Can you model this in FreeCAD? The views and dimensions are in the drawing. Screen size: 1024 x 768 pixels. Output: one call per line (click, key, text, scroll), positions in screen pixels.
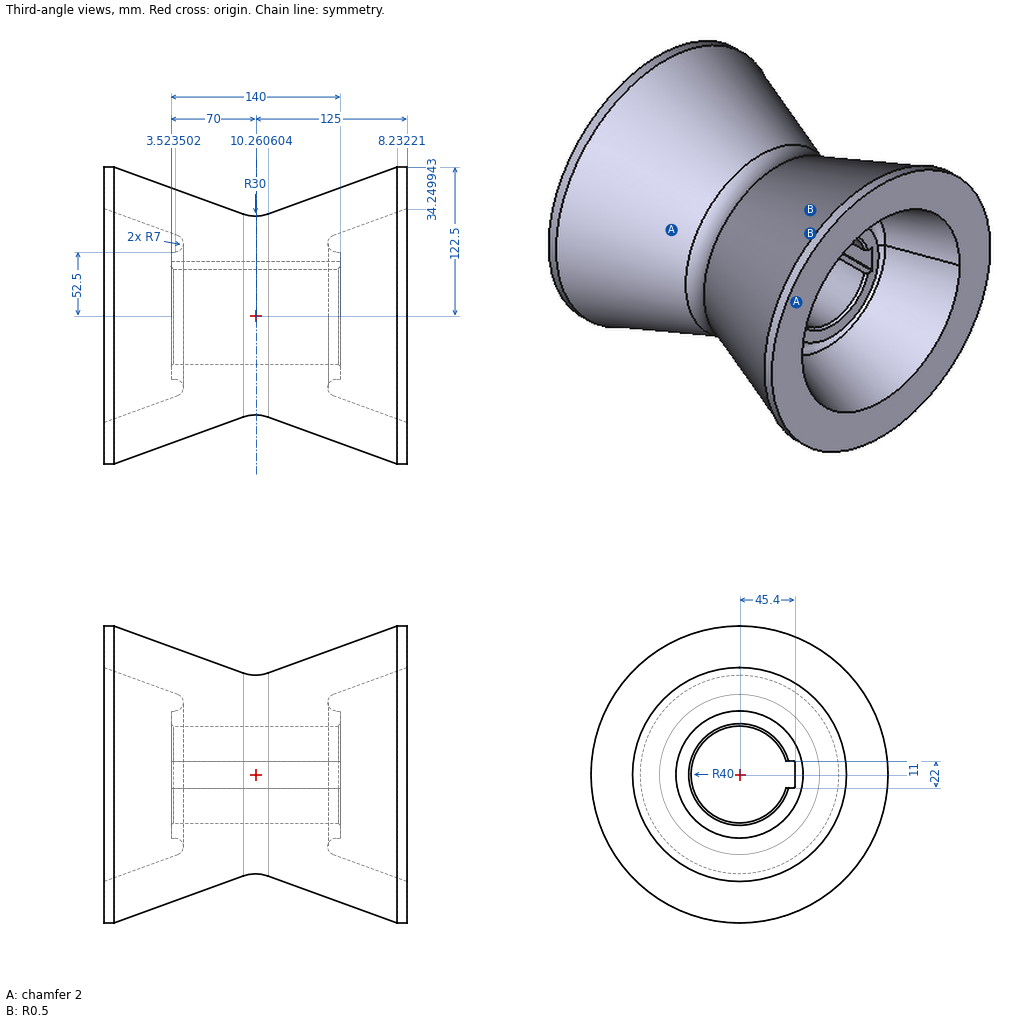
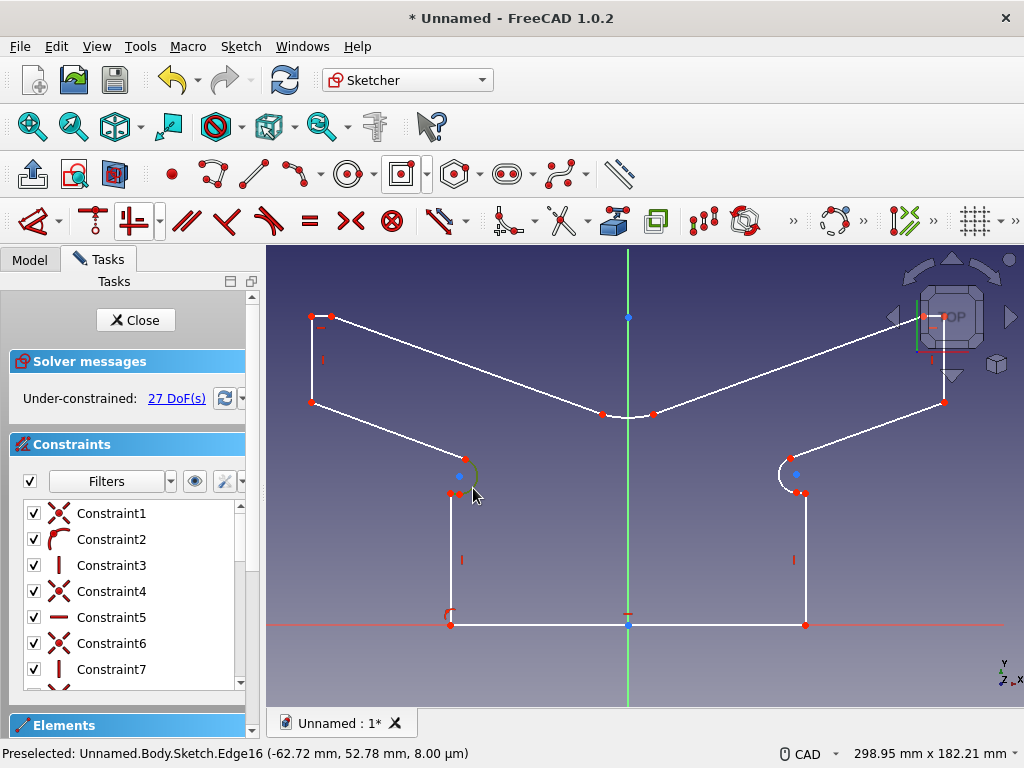
click(269, 222)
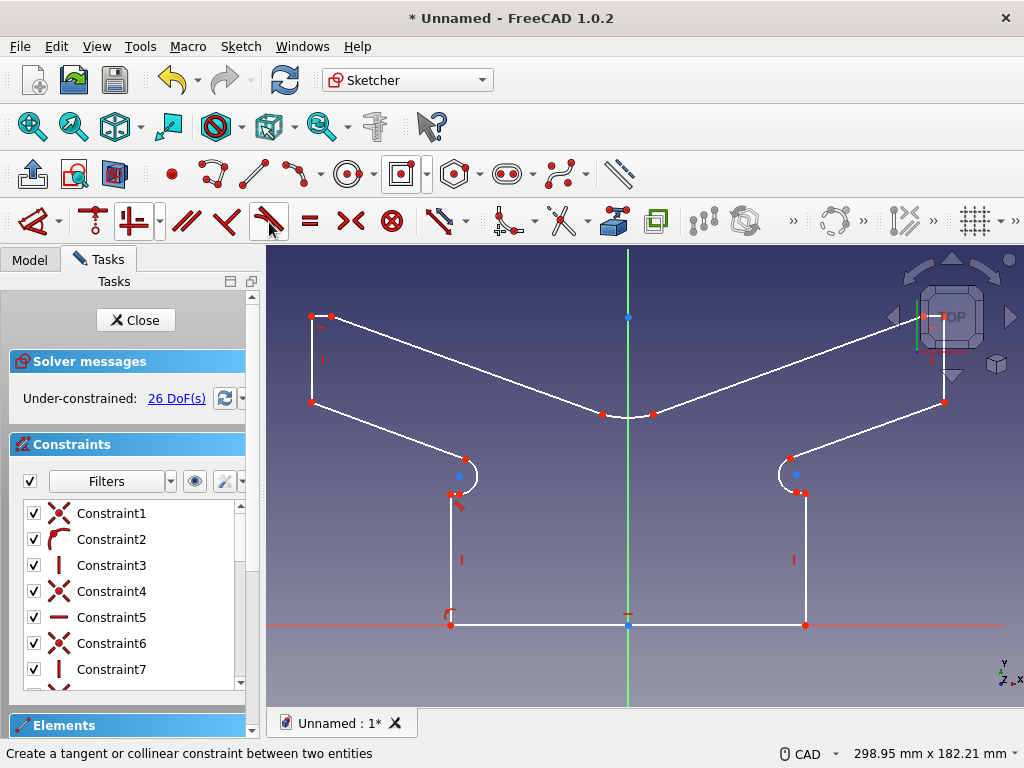
scroll(801, 493, up, 6)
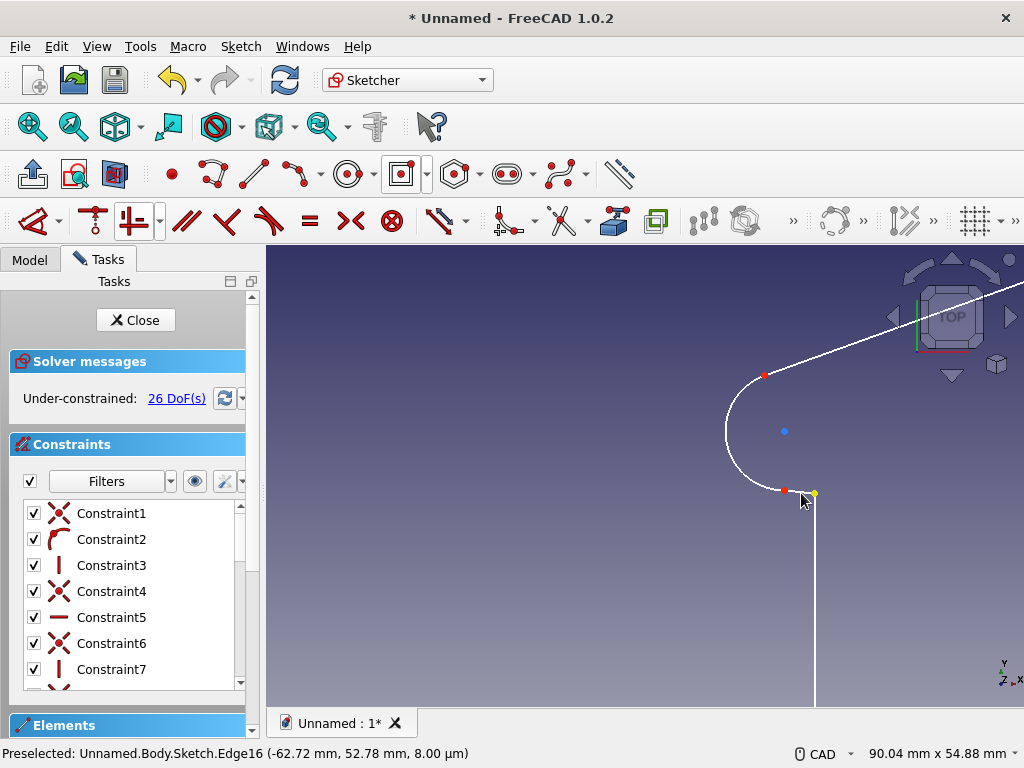
click(800, 492)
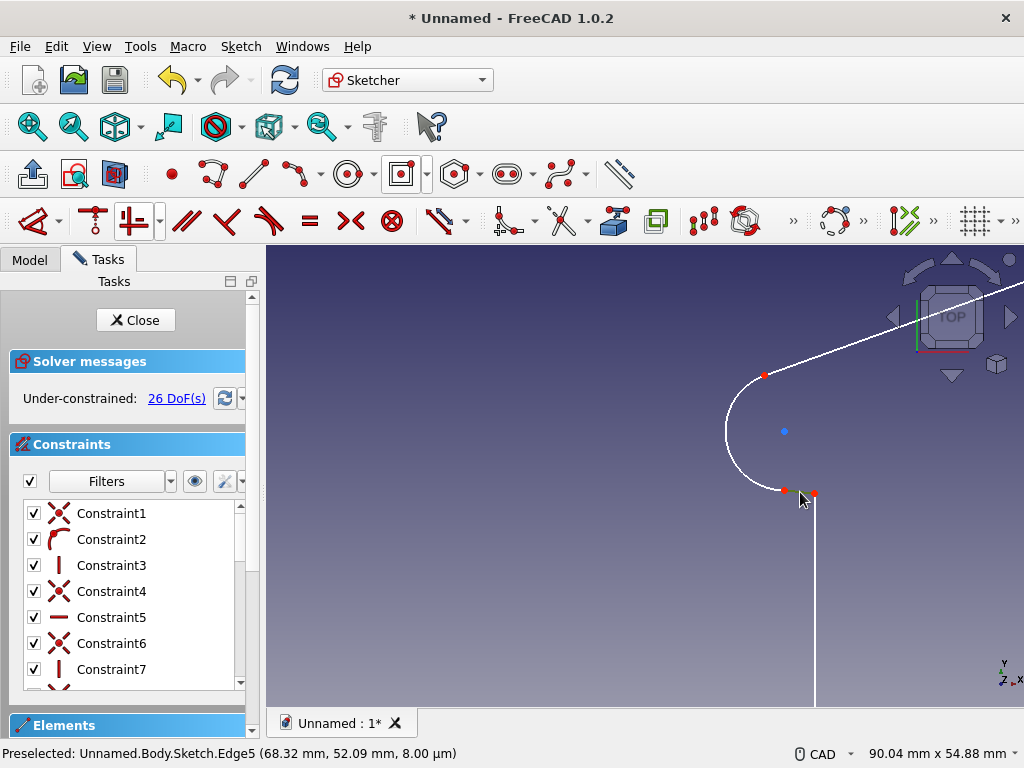
scroll(665, 491, down, 8)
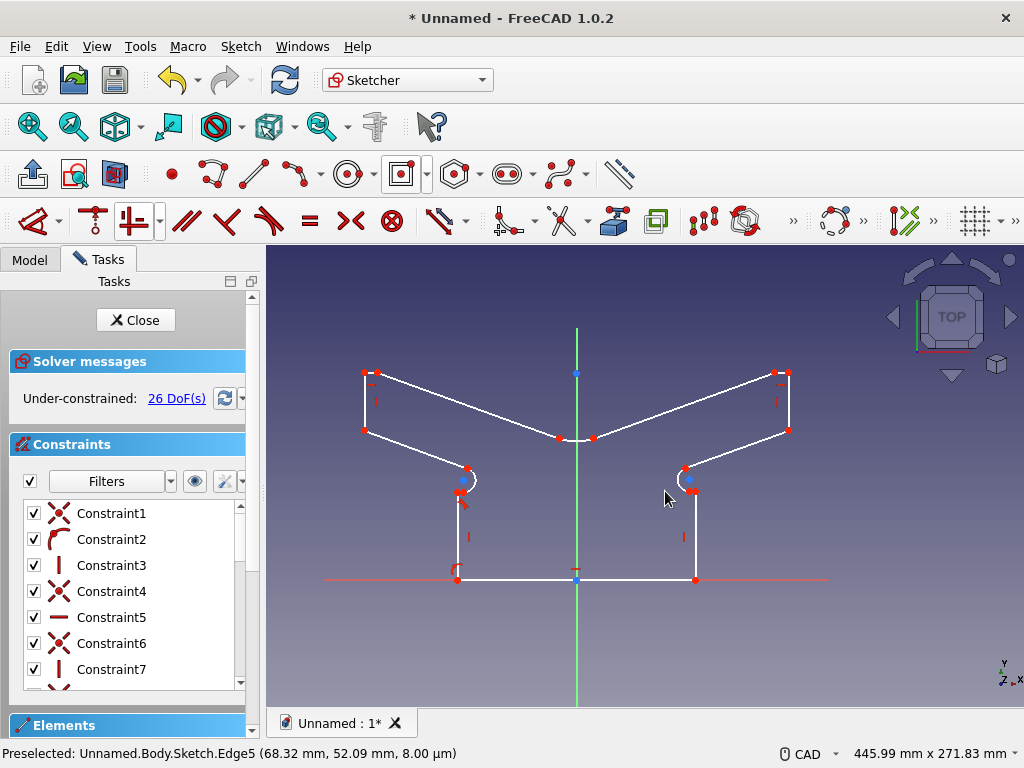
scroll(679, 475, up, 2)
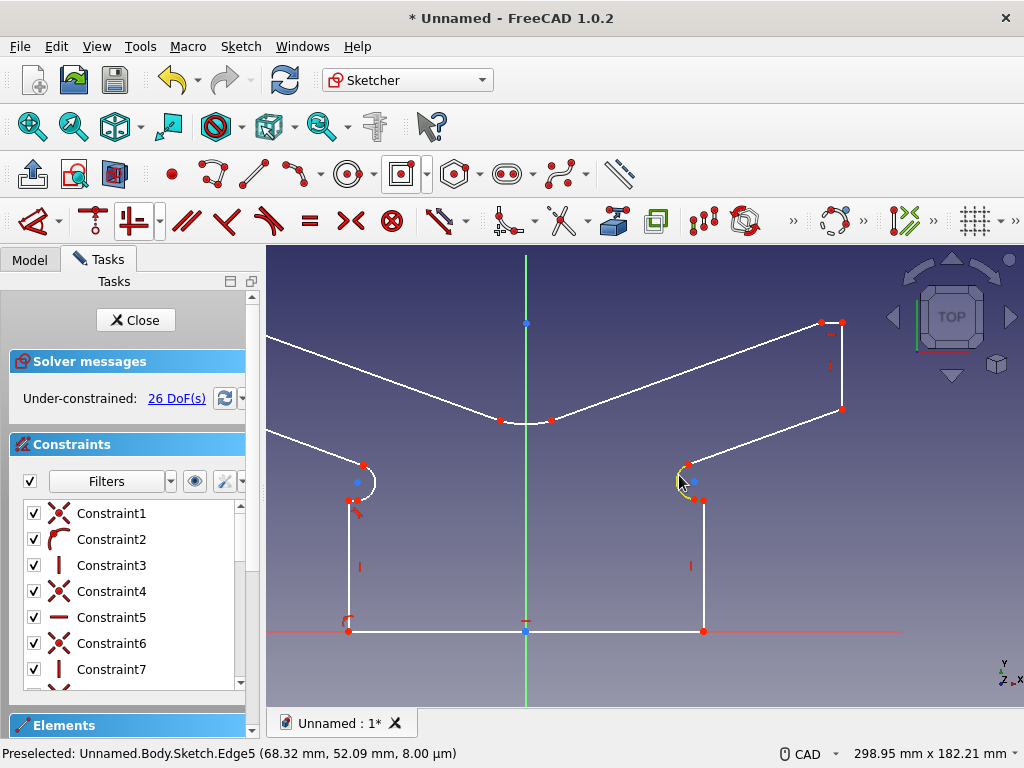
click(678, 475)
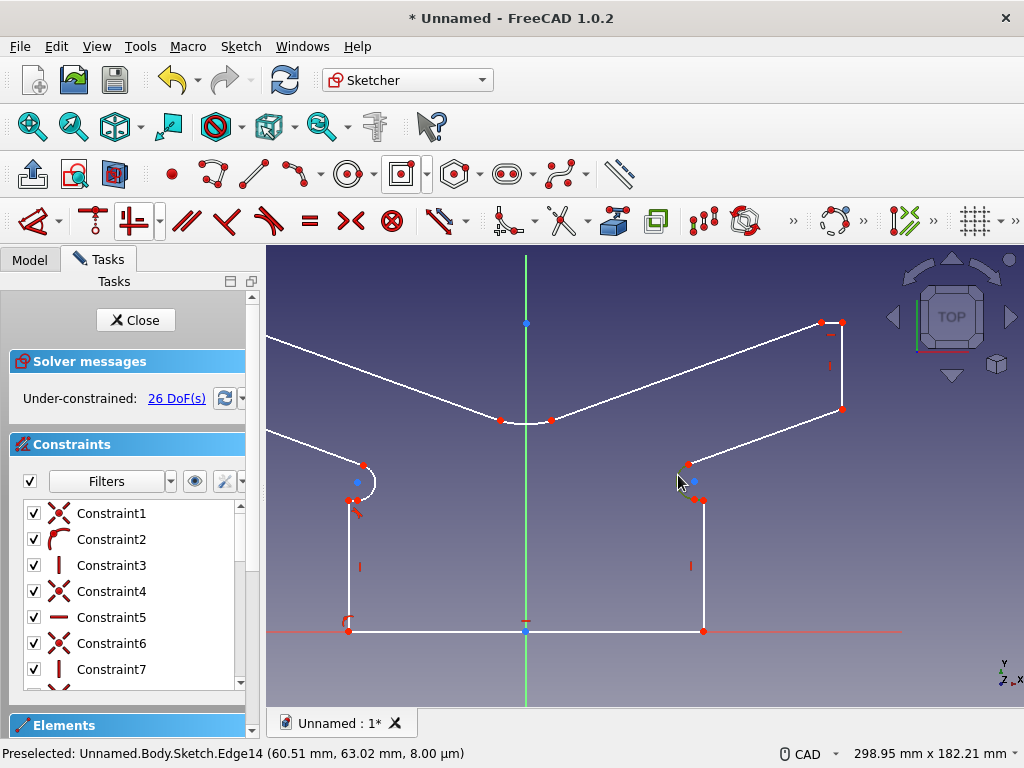
click(269, 222)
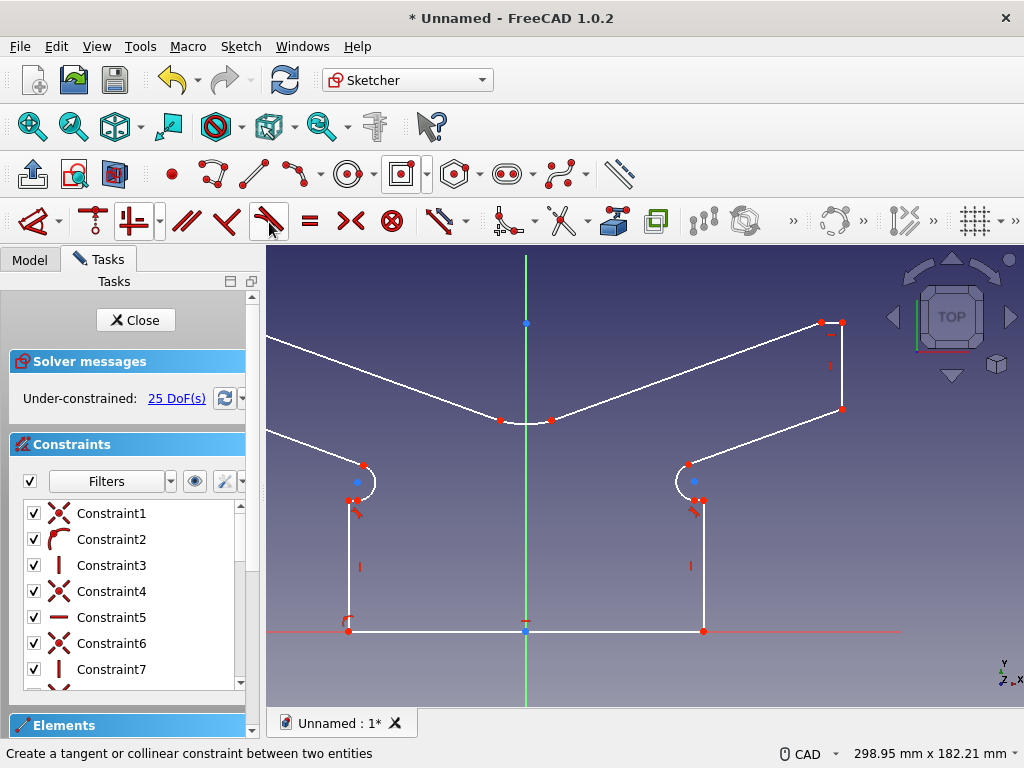
click(735, 448)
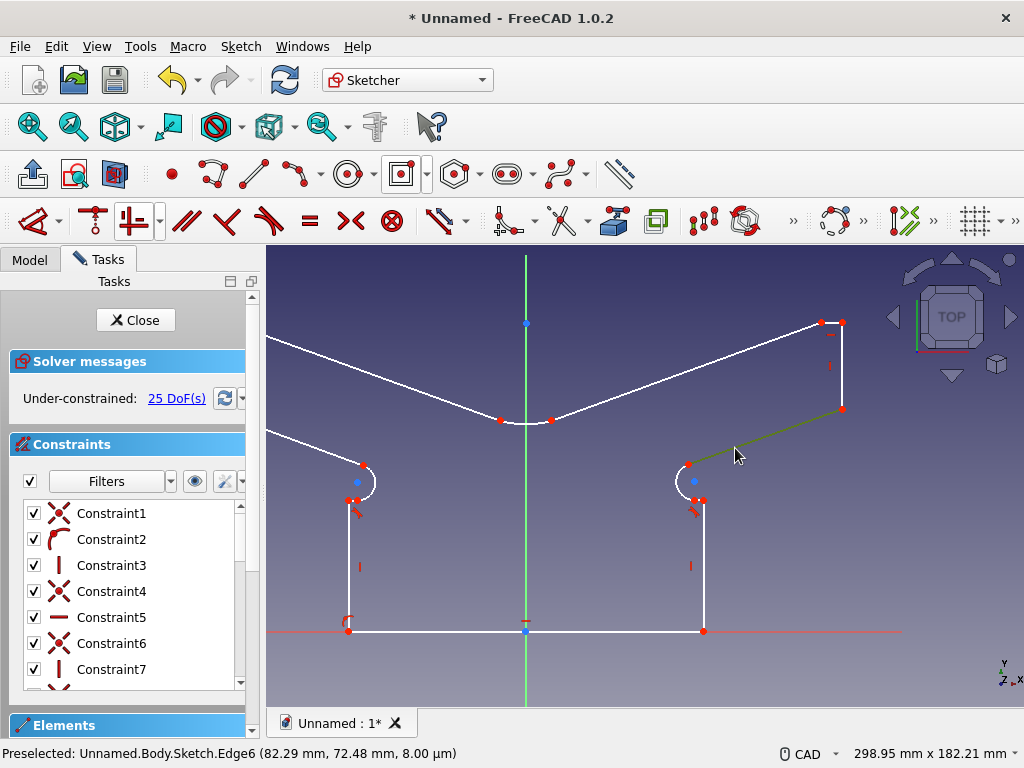
click(678, 475)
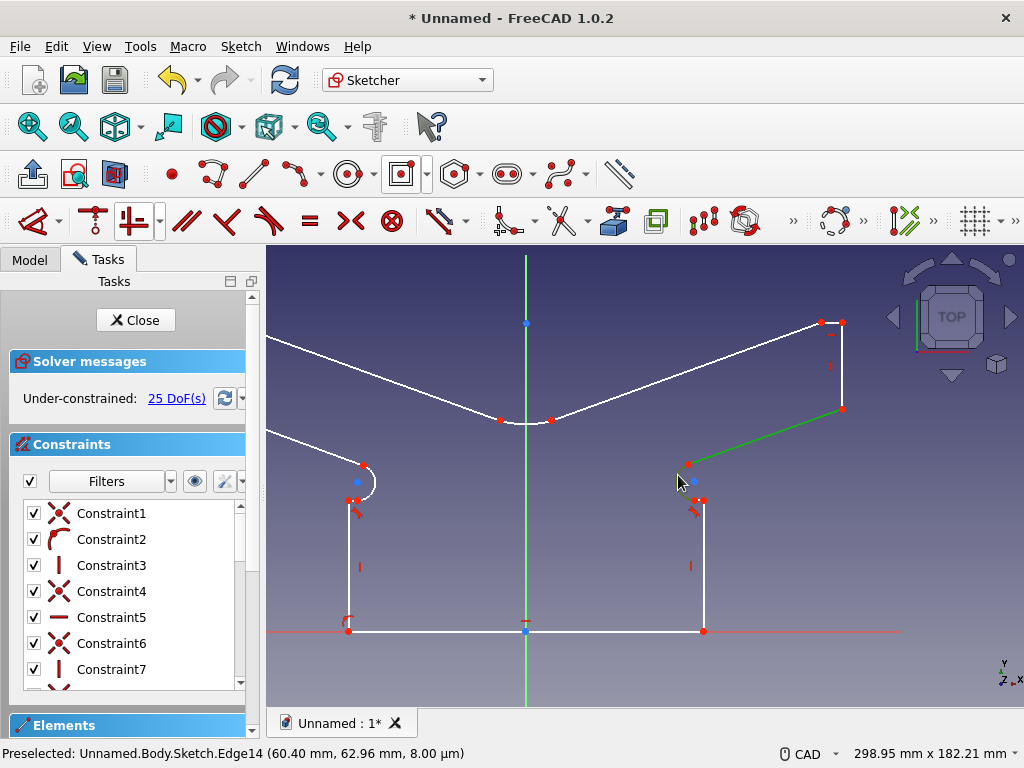
click(269, 222)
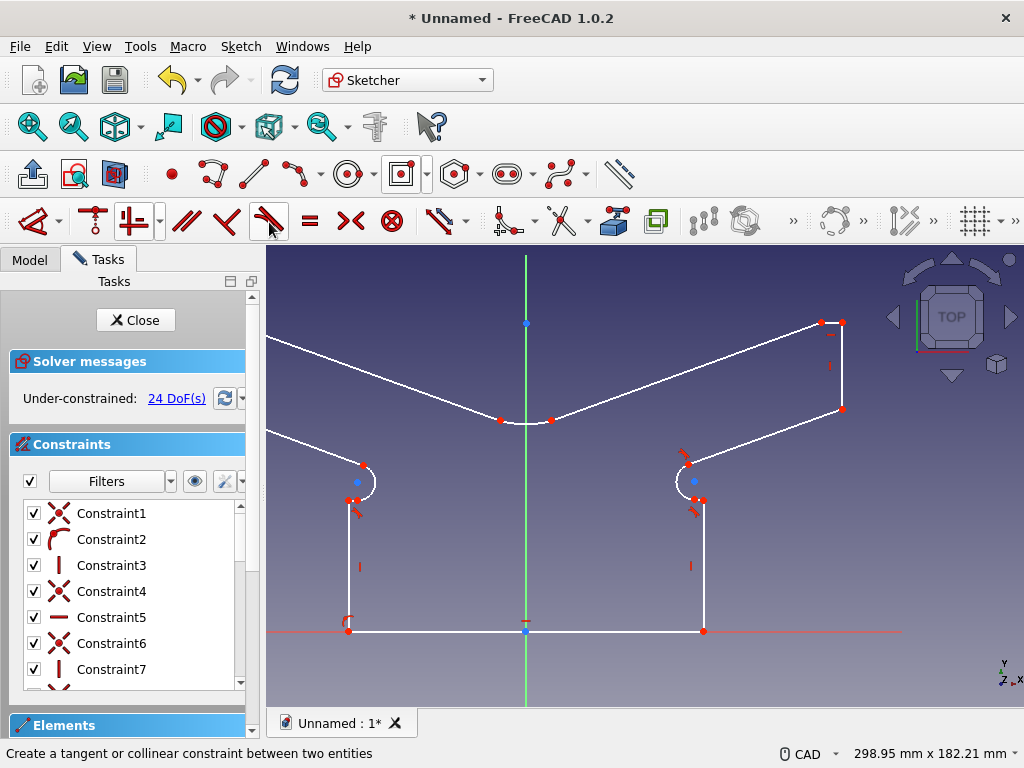
click(740, 352)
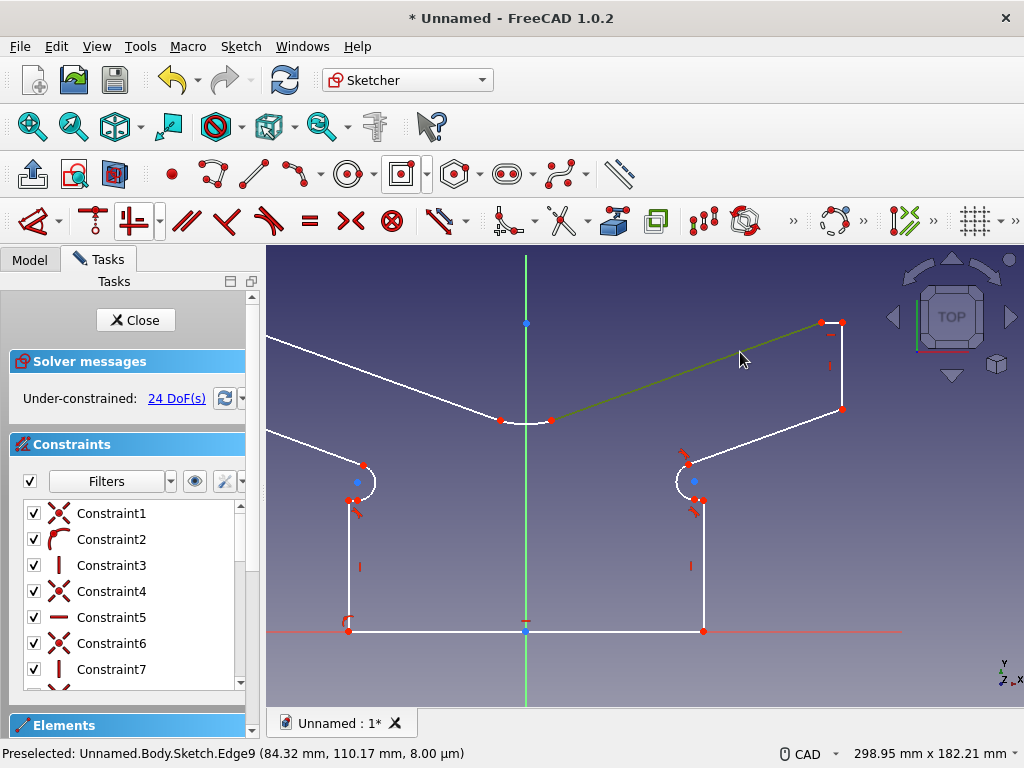
scroll(516, 424, up, 2)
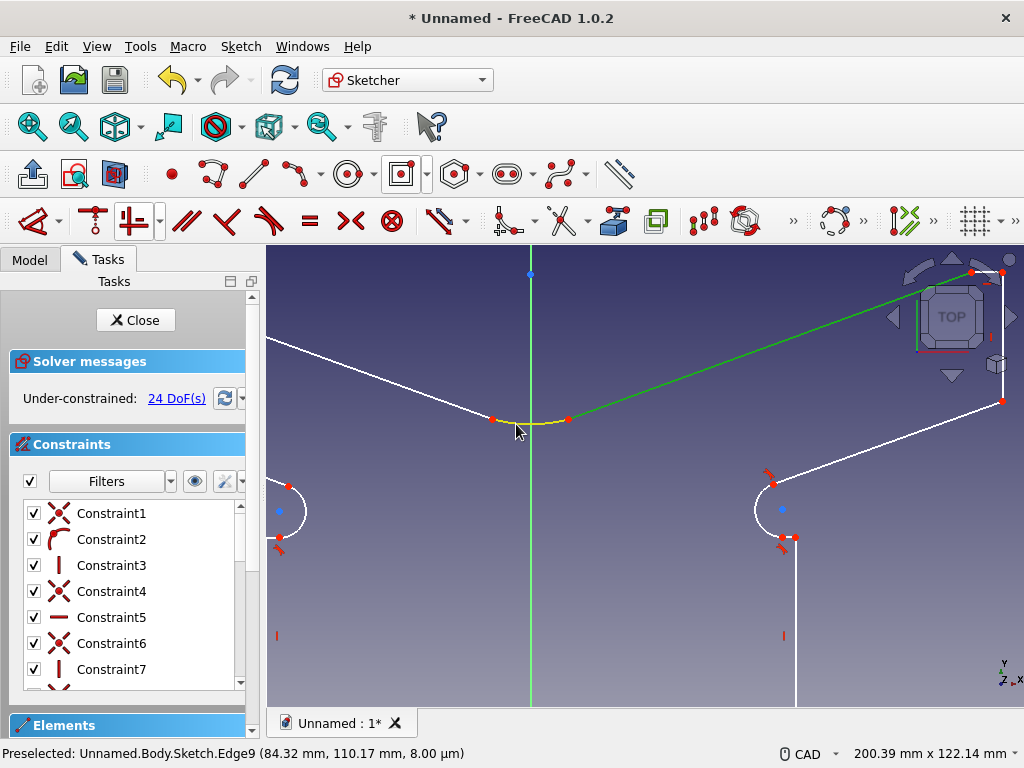
click(516, 423)